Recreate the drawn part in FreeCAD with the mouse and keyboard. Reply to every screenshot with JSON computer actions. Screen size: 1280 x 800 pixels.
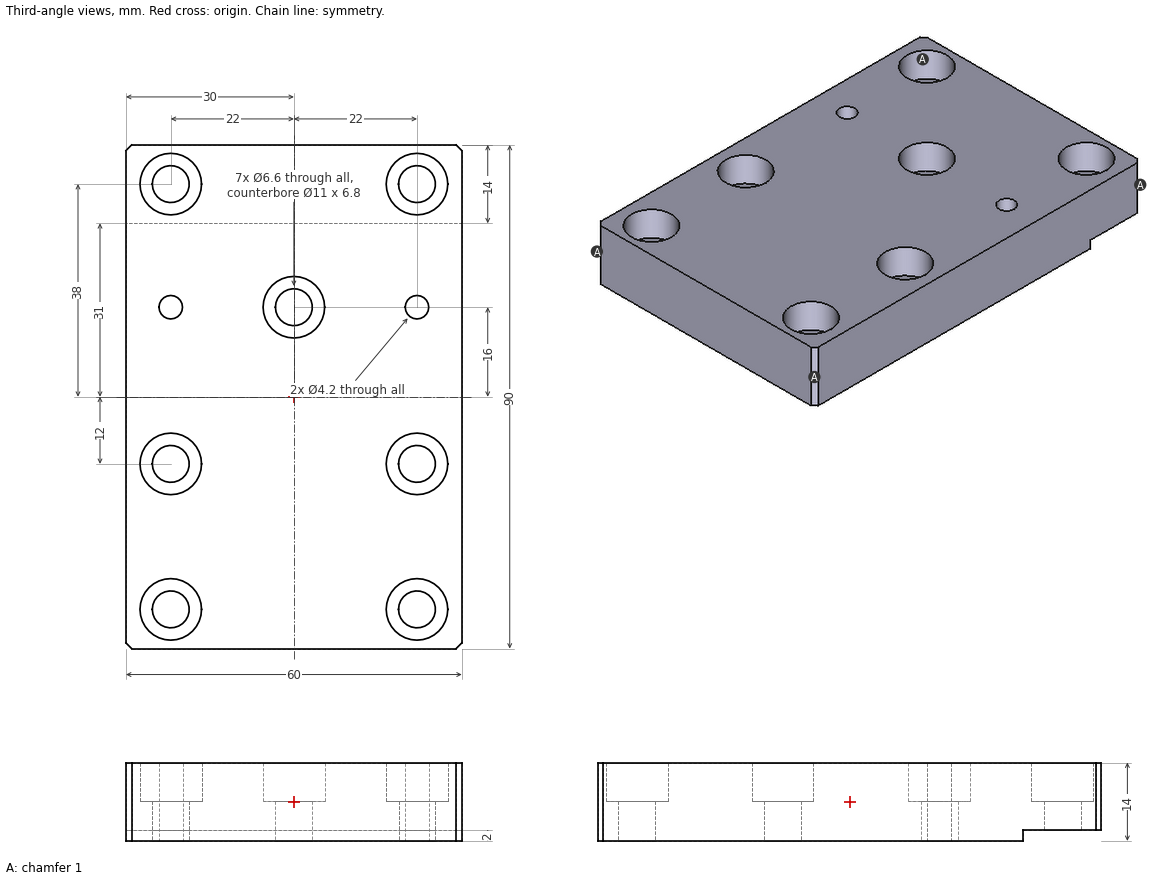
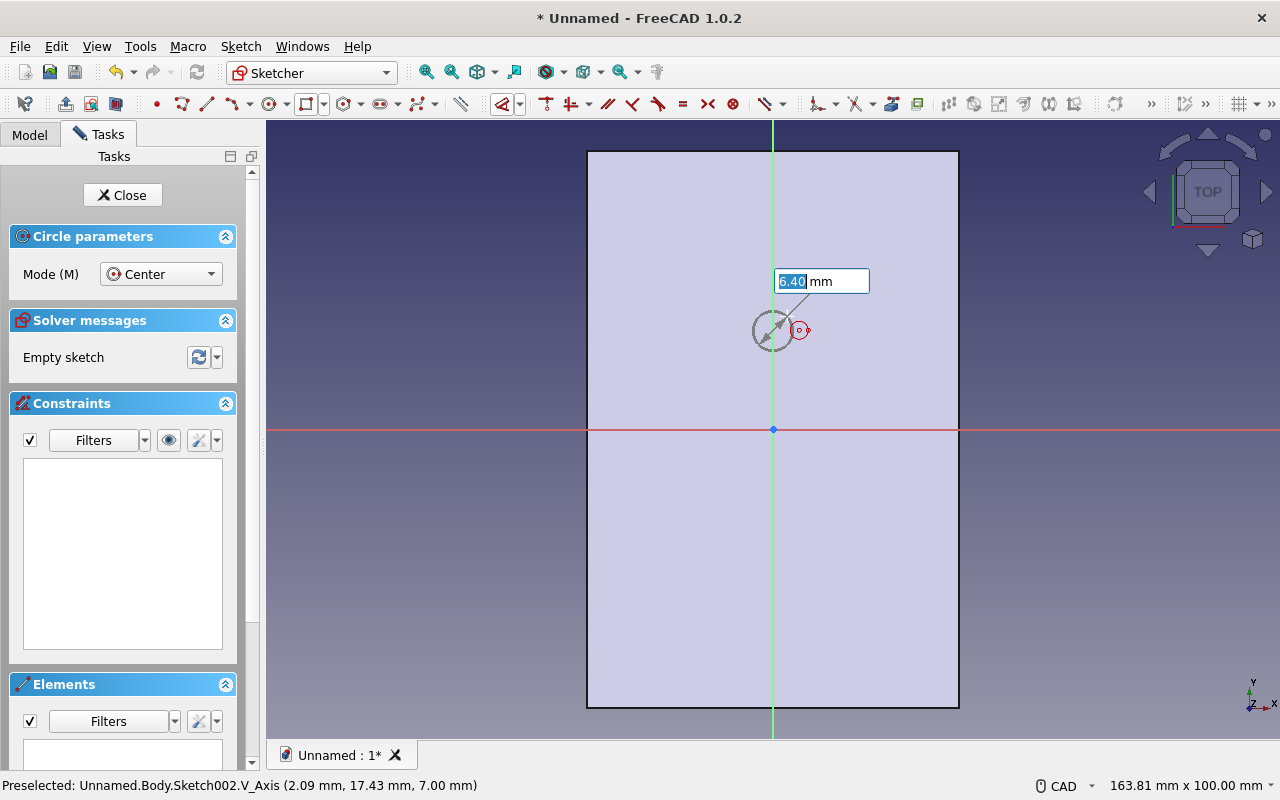
{"action": "type", "text": "6.6"}
{"action": "key", "text": "Return"}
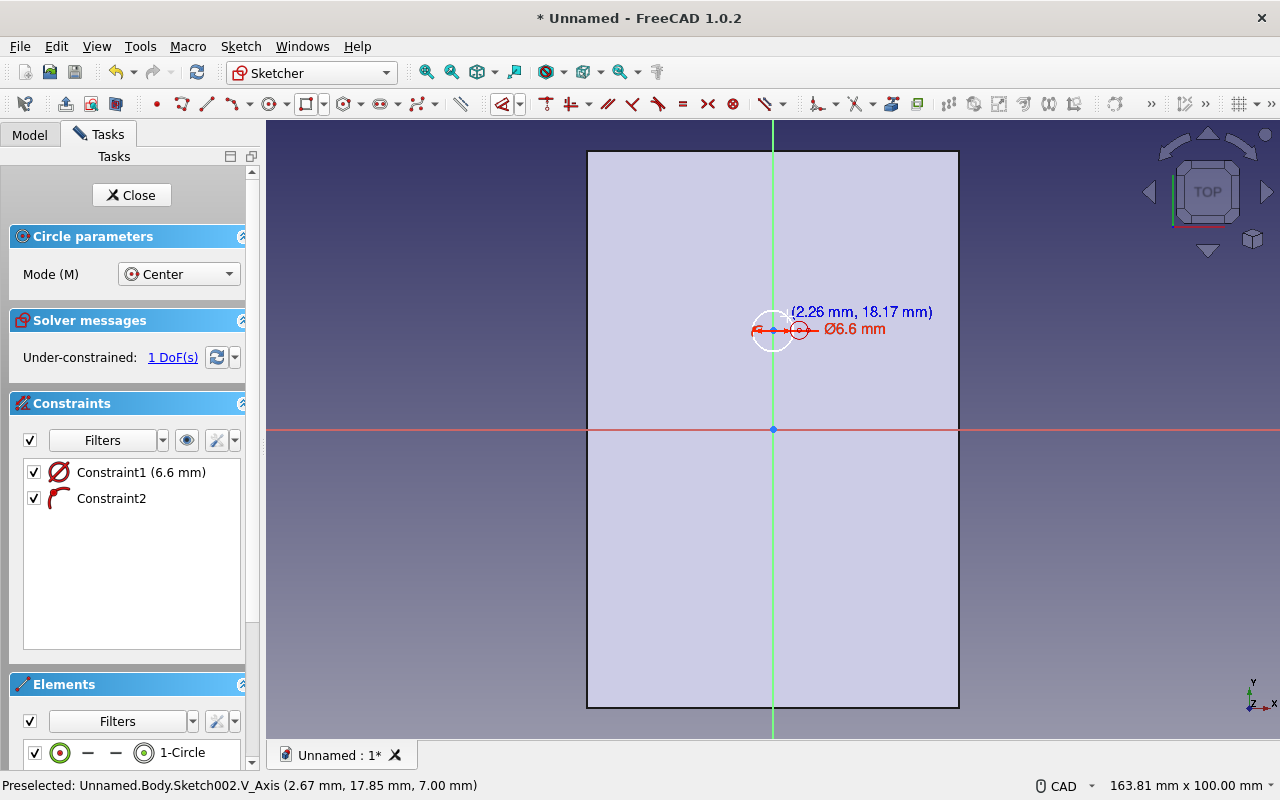
{"action": "left_click", "coordinate": [637, 194]}
{"action": "mouse_move", "coordinate": [651, 180]}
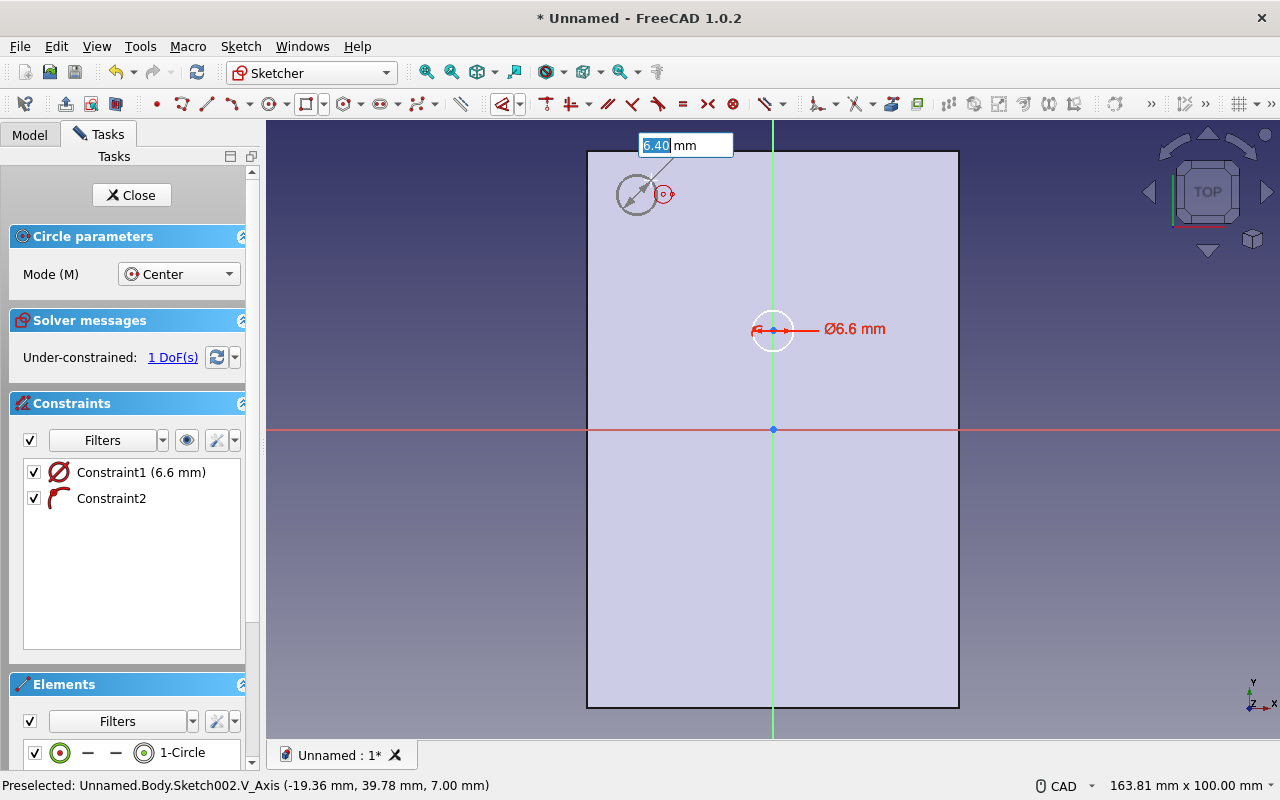
{"action": "type", "text": "6.6"}
{"action": "key", "text": "Return"}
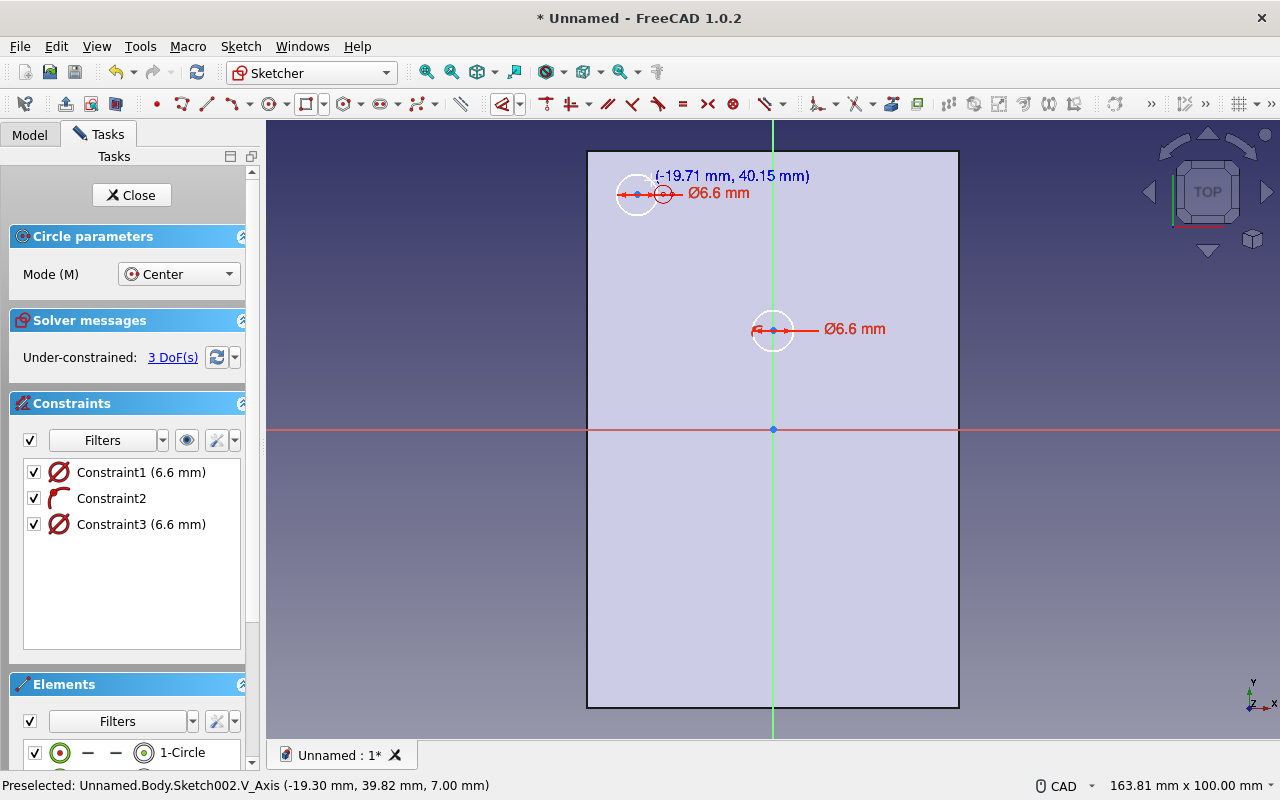
{"action": "left_click", "coordinate": [909, 194]}
{"action": "mouse_move", "coordinate": [924, 180]}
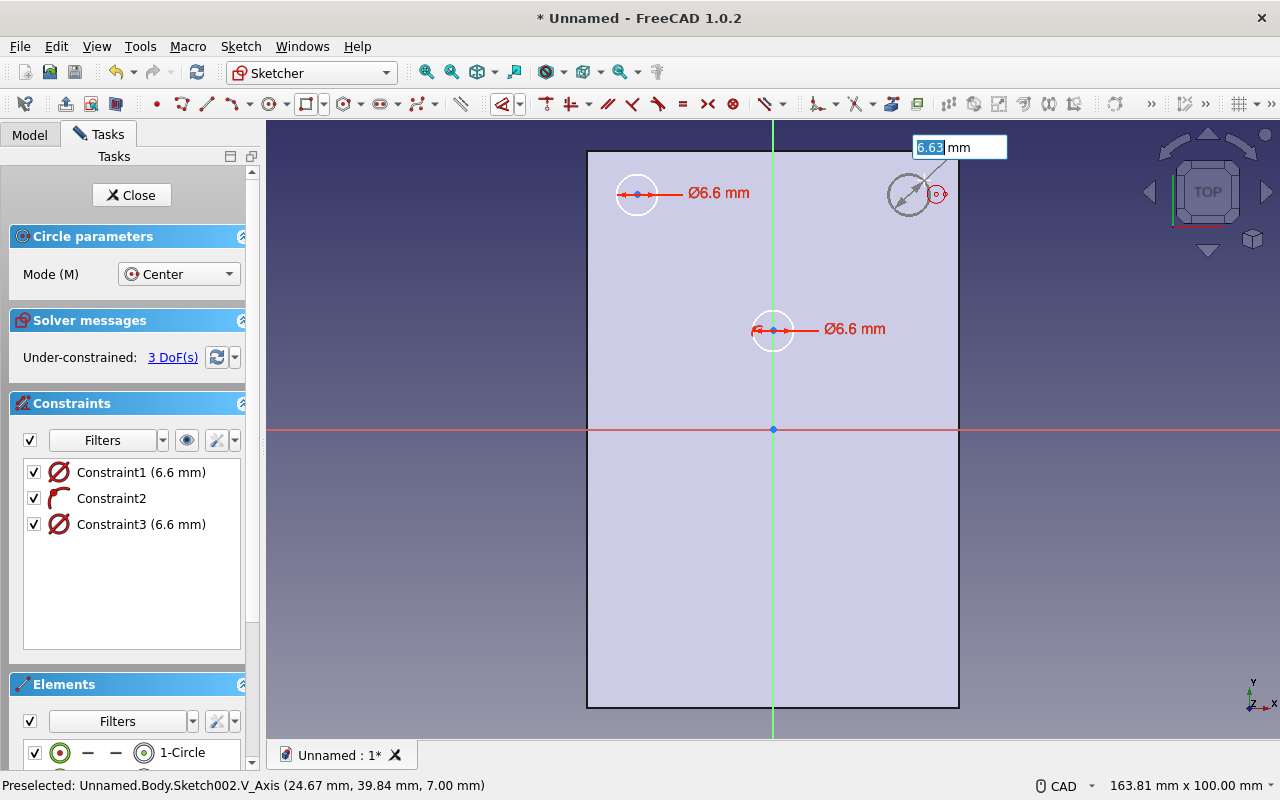
{"action": "type", "text": "6.6"}
{"action": "key", "text": "Return"}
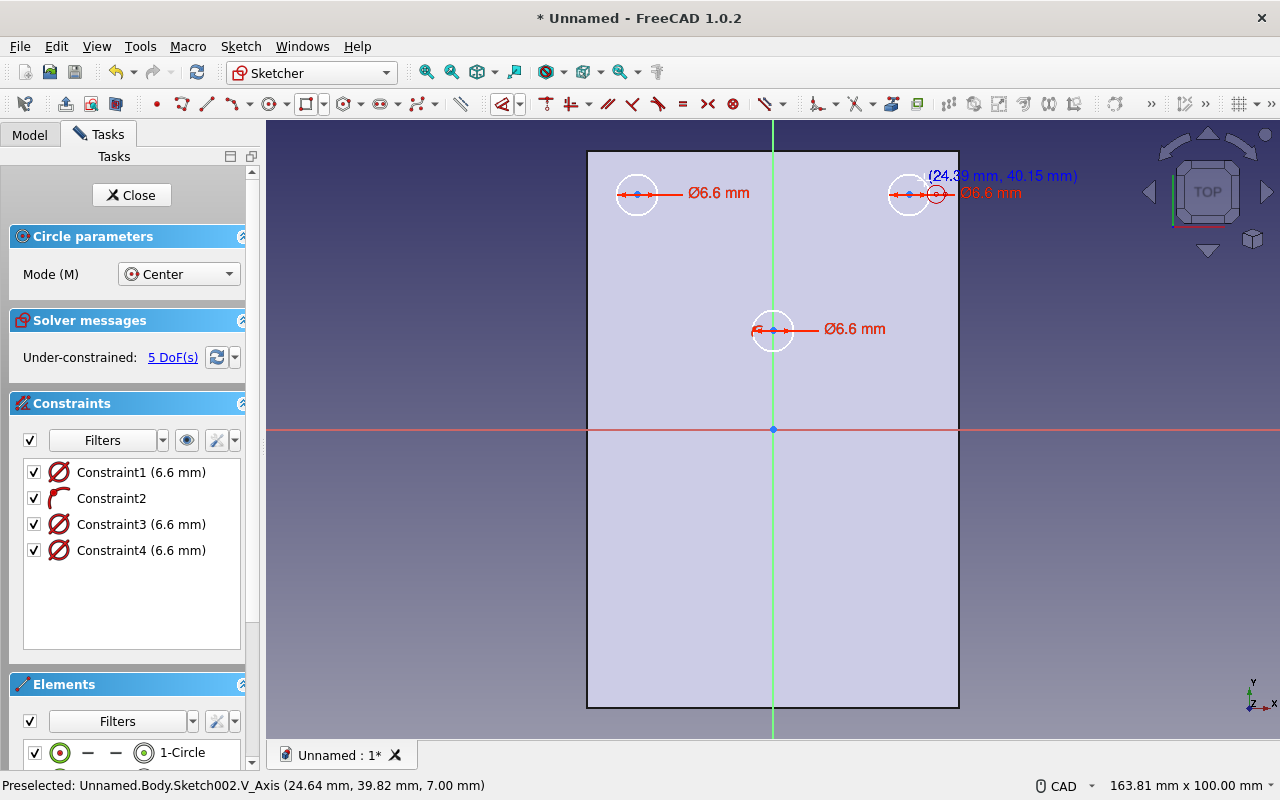
{"action": "left_click", "coordinate": [637, 504]}
{"action": "mouse_move", "coordinate": [651, 489]}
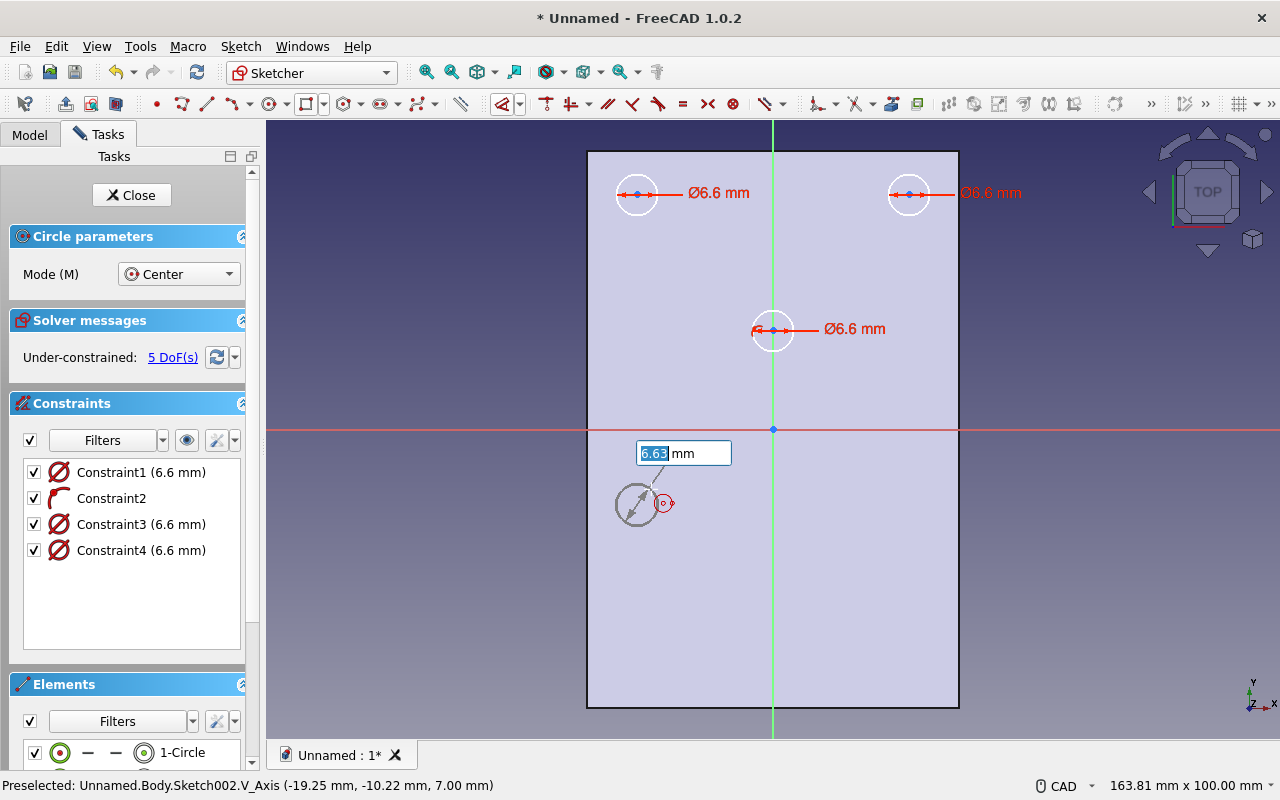
{"action": "type", "text": "6.6"}
{"action": "key", "text": "Return"}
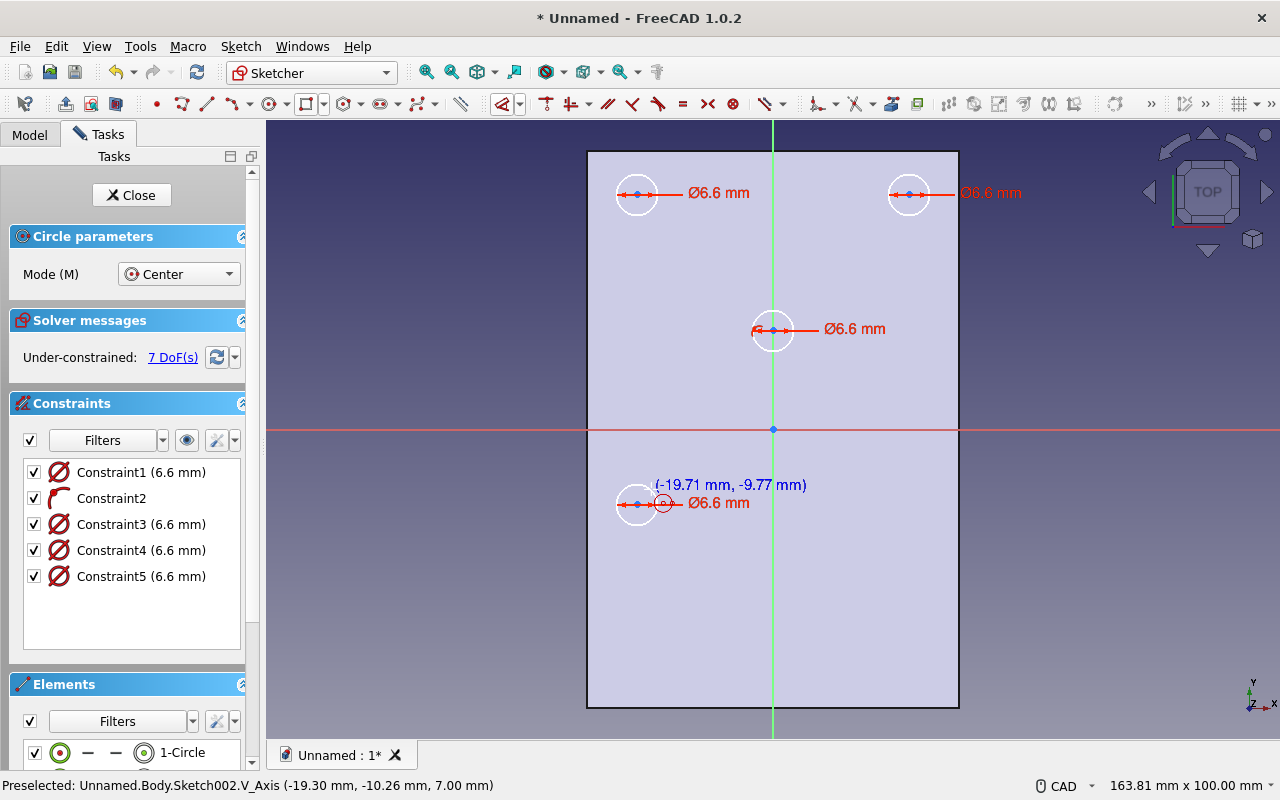
{"action": "left_click", "coordinate": [909, 665]}
{"action": "mouse_move", "coordinate": [924, 650]}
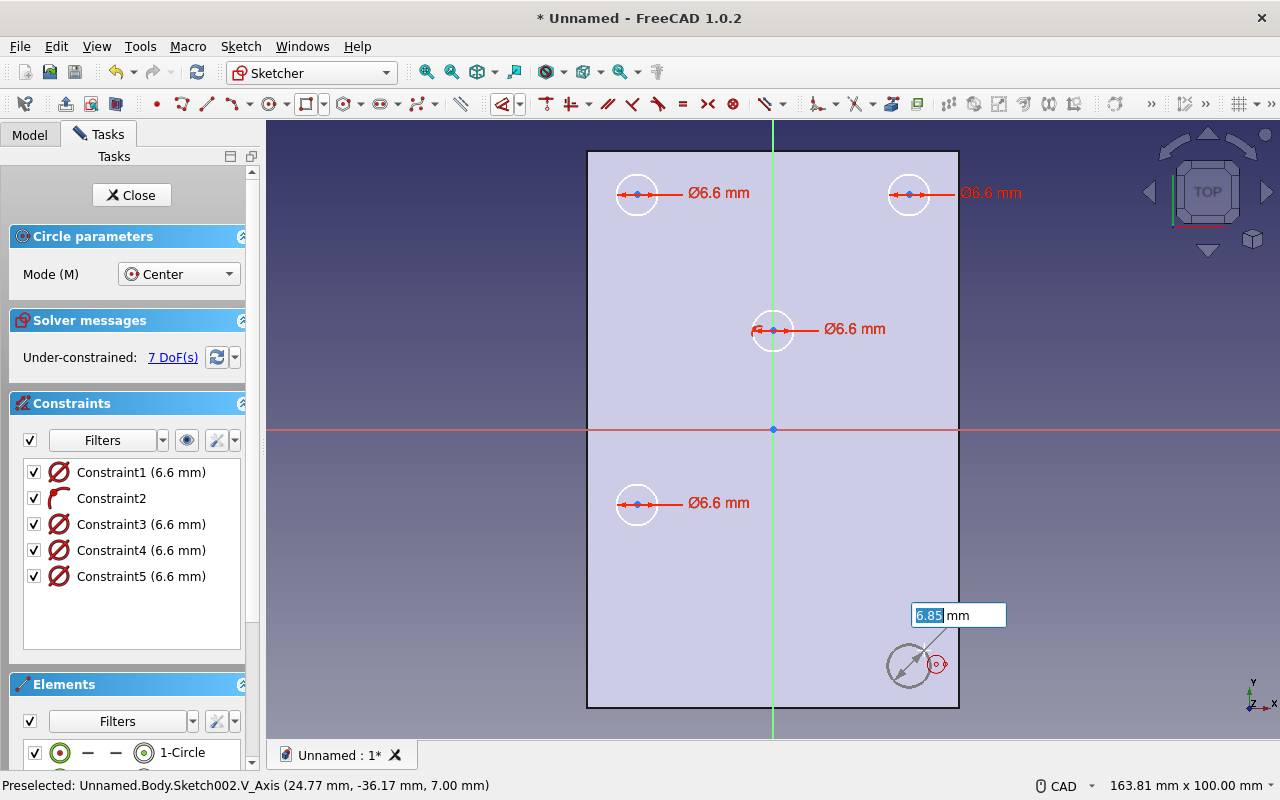
{"action": "type", "text": "6.6"}
{"action": "key", "text": "Return"}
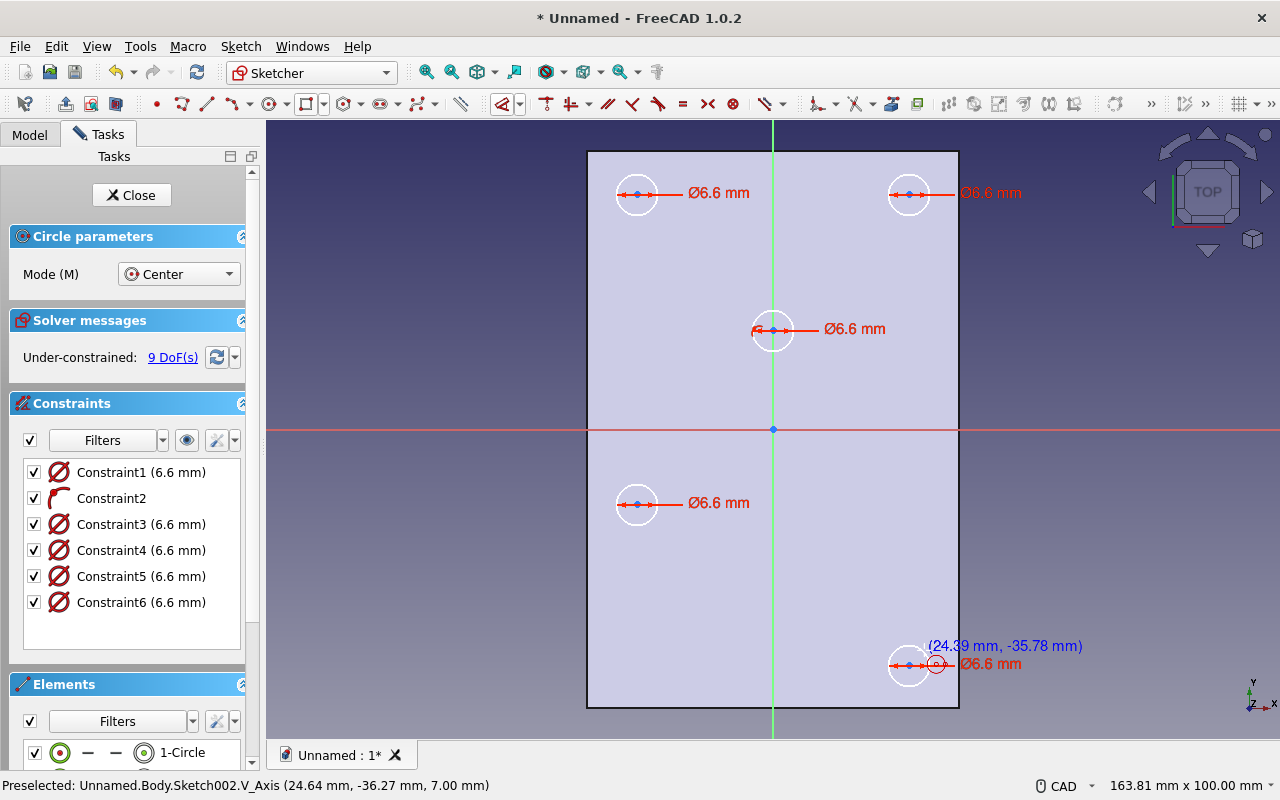
{"action": "left_click", "coordinate": [637, 665]}
{"action": "mouse_move", "coordinate": [651, 650]}